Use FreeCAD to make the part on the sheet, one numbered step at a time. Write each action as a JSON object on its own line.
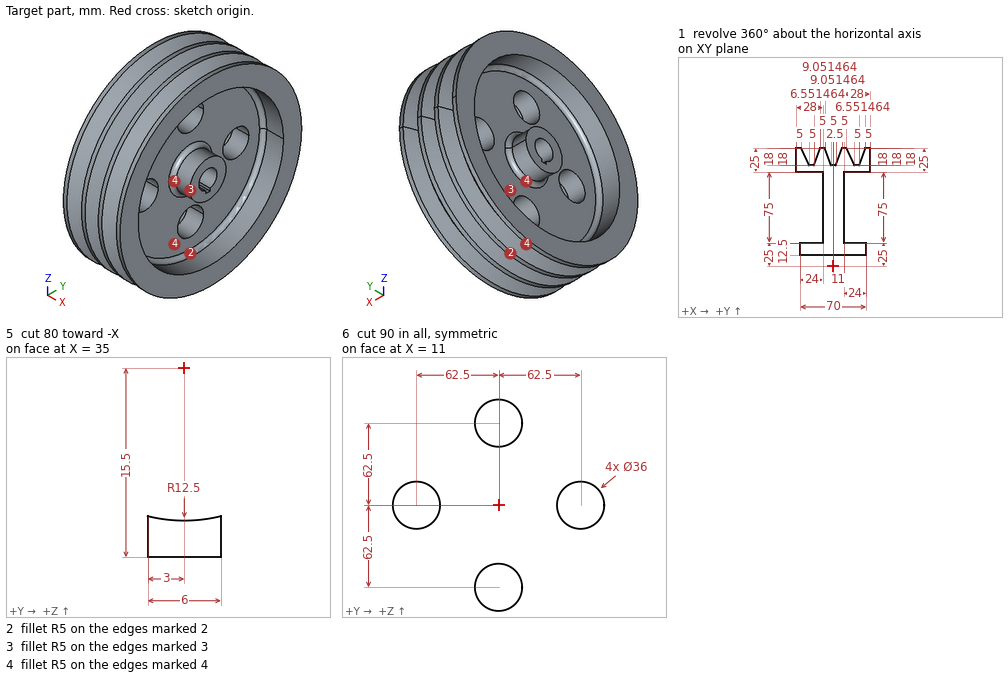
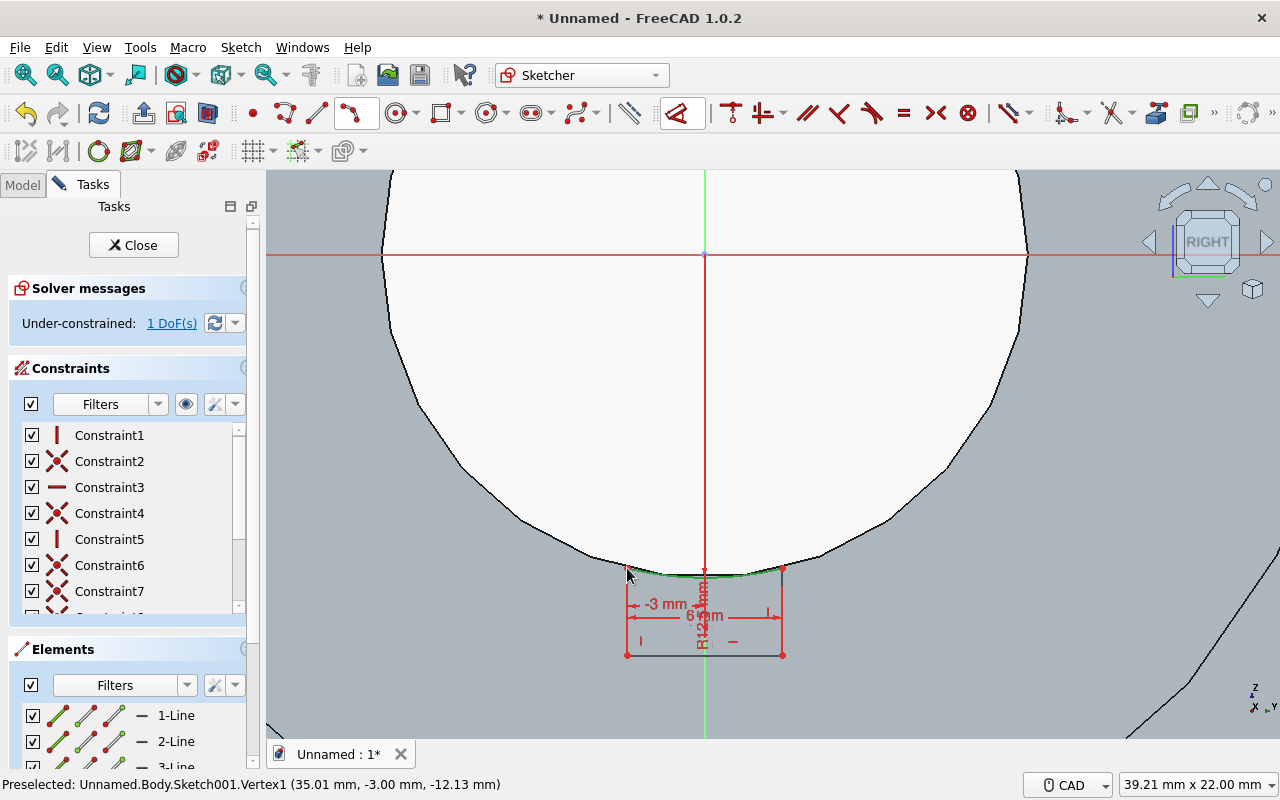
{"action": "left_click", "coordinate": [627, 656]}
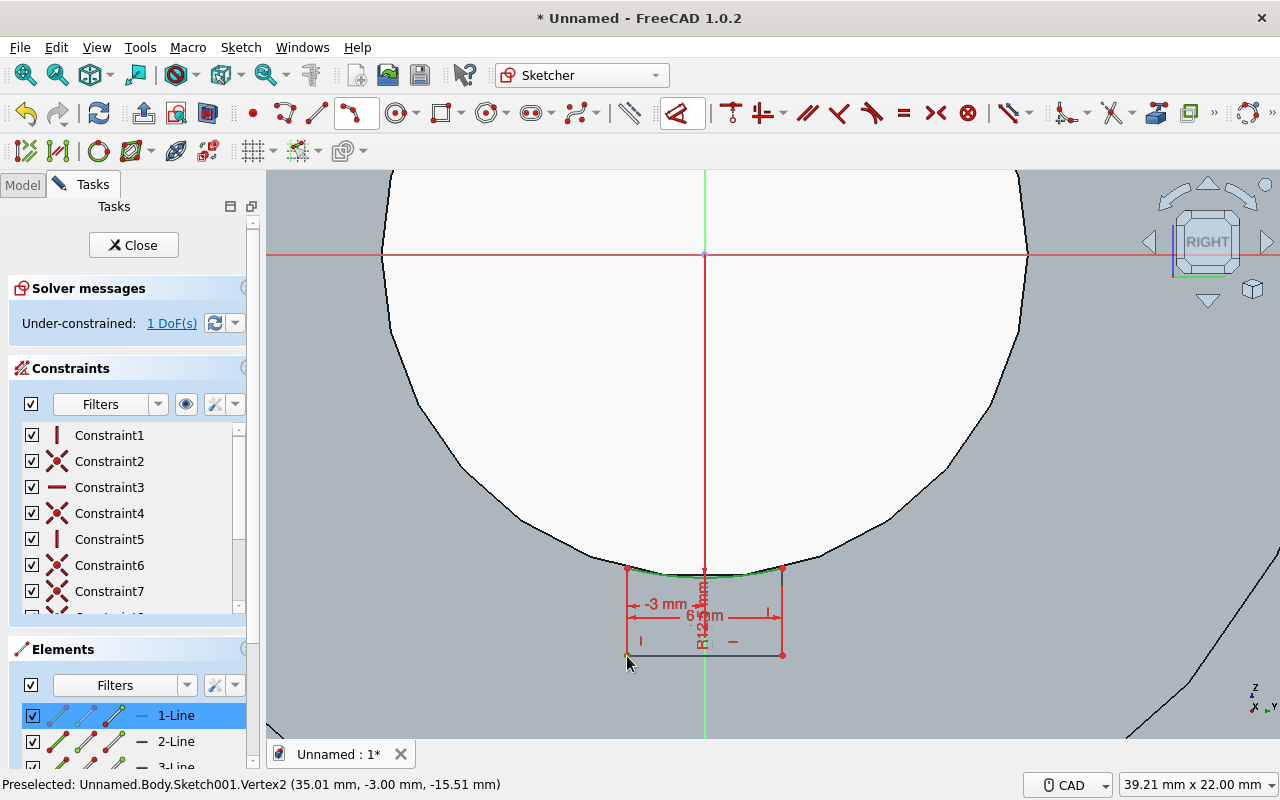
{"action": "left_click", "coordinate": [700, 114]}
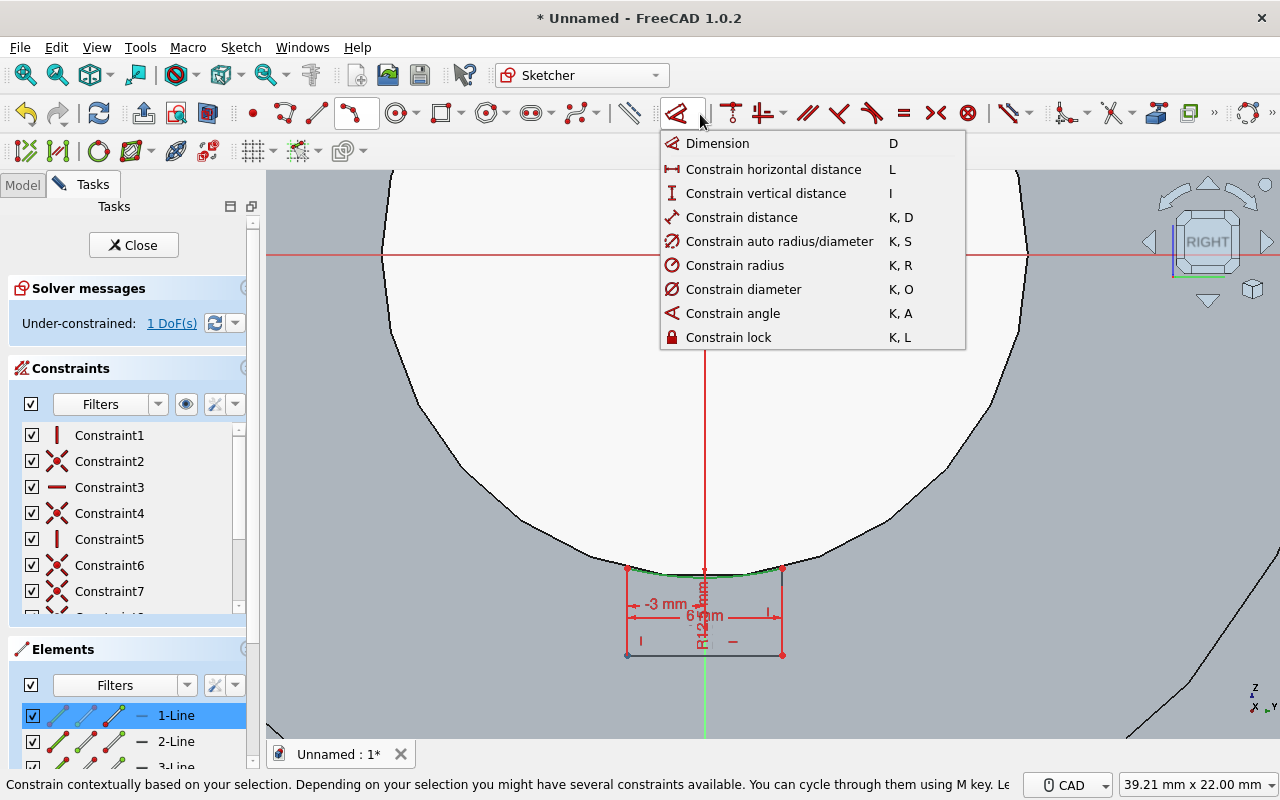
{"action": "left_click", "coordinate": [813, 193]}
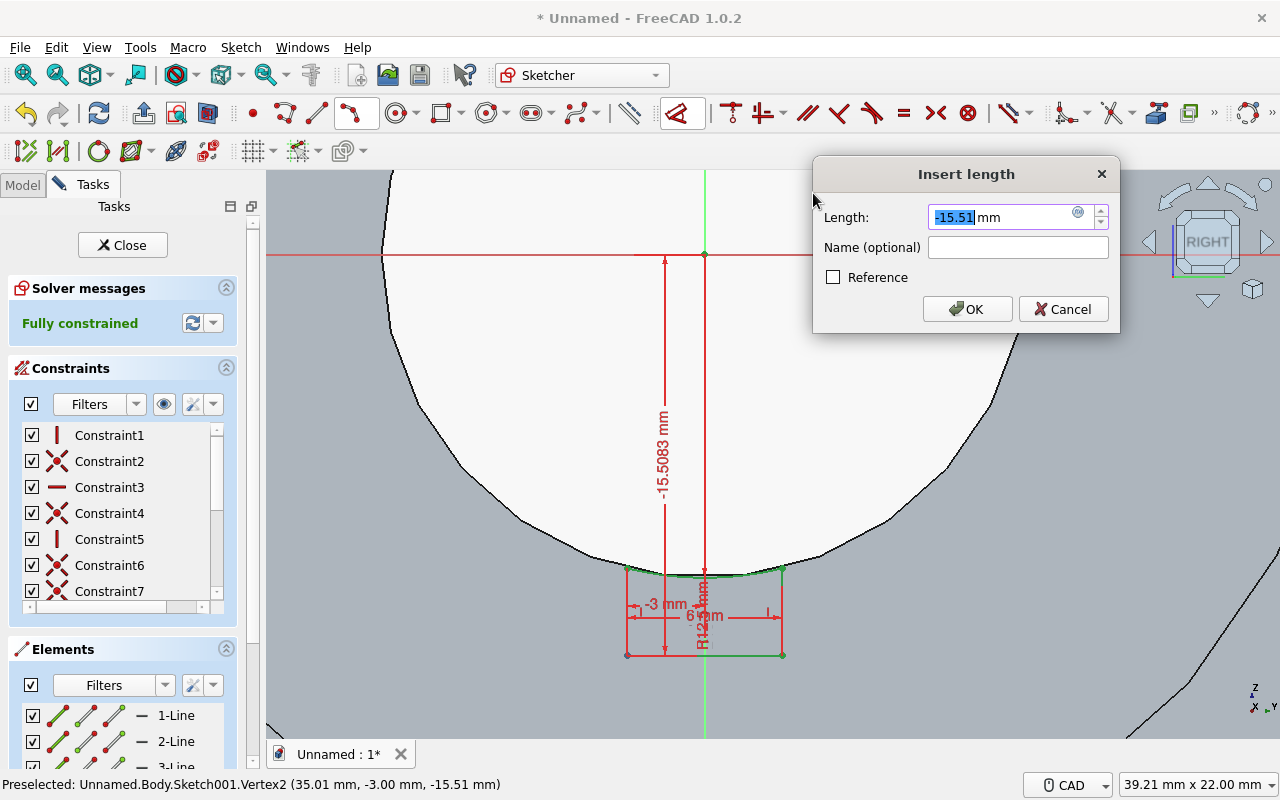
{"action": "type", "text": "-15.5"}
{"action": "key", "text": "Return"}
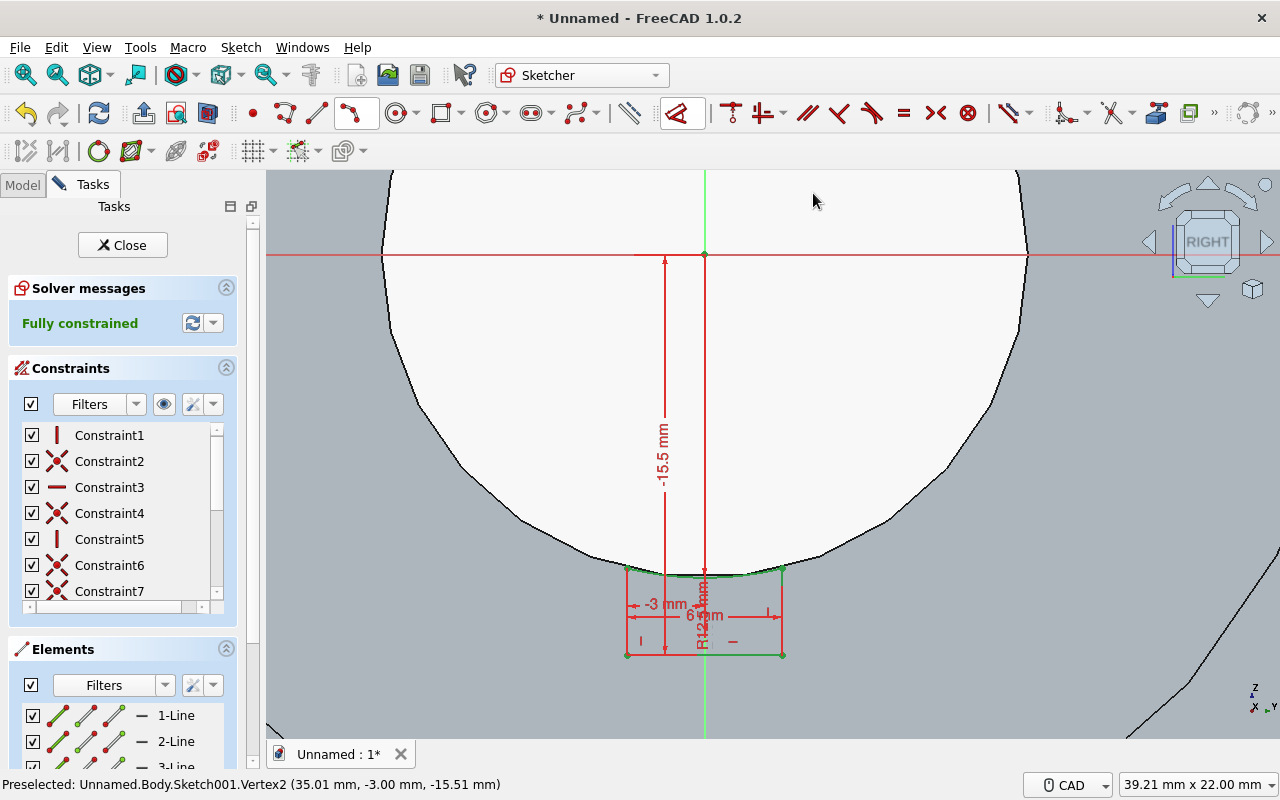
{"action": "left_click", "coordinate": [123, 245]}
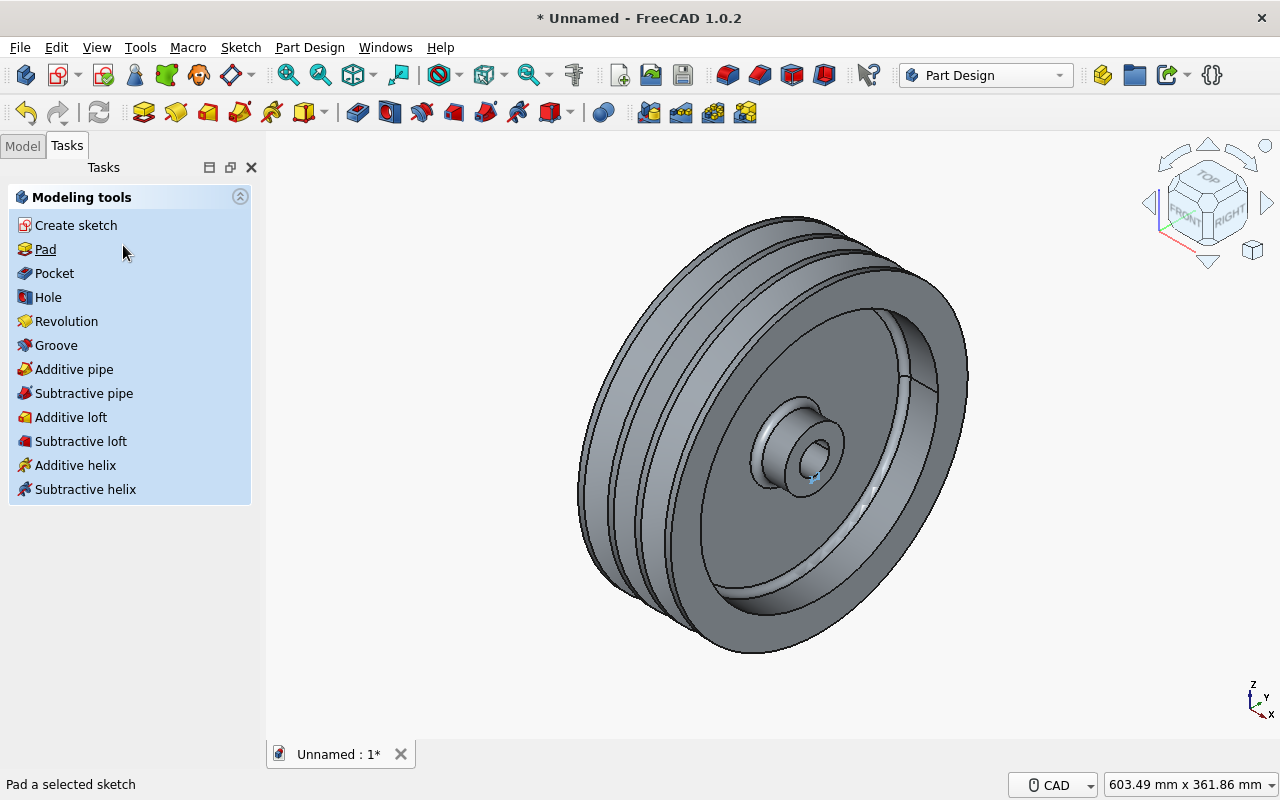
{"action": "left_click", "coordinate": [358, 112]}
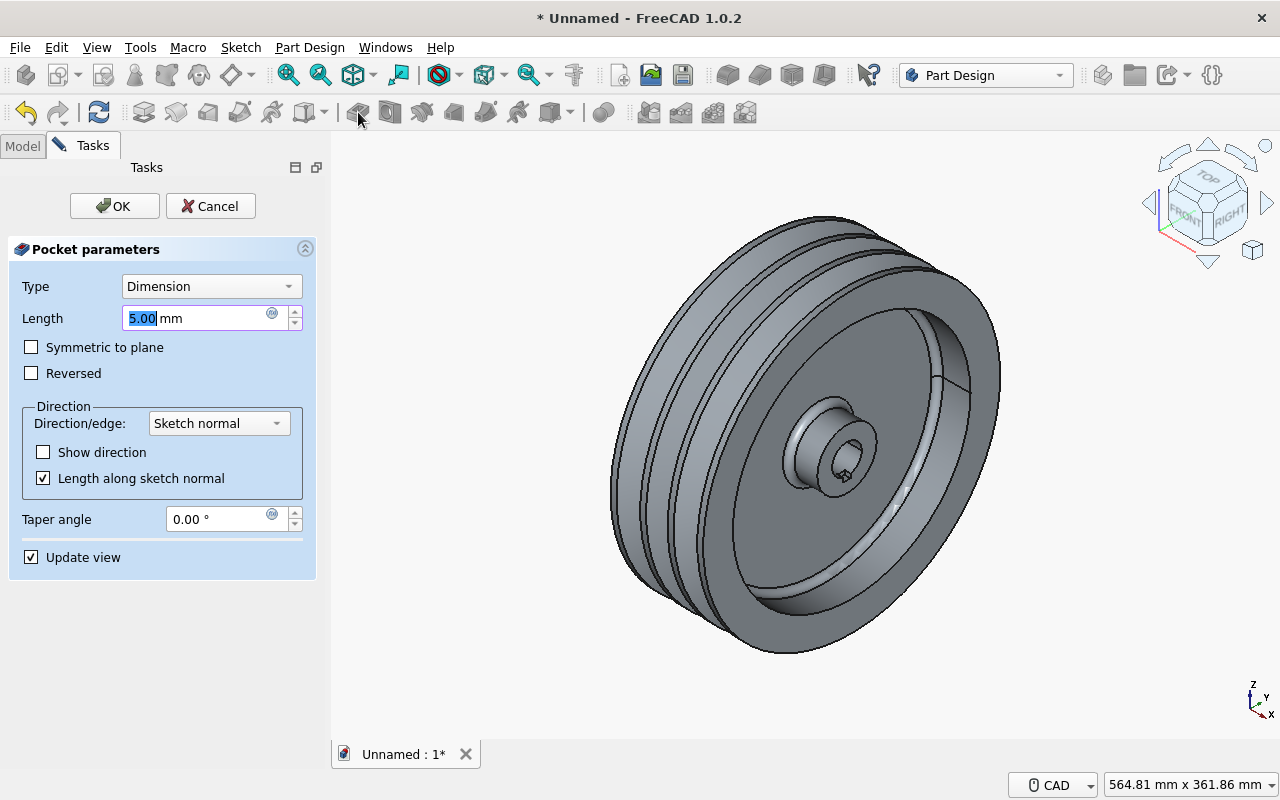
{"action": "type", "text": "80"}
{"action": "key", "text": "Tab"}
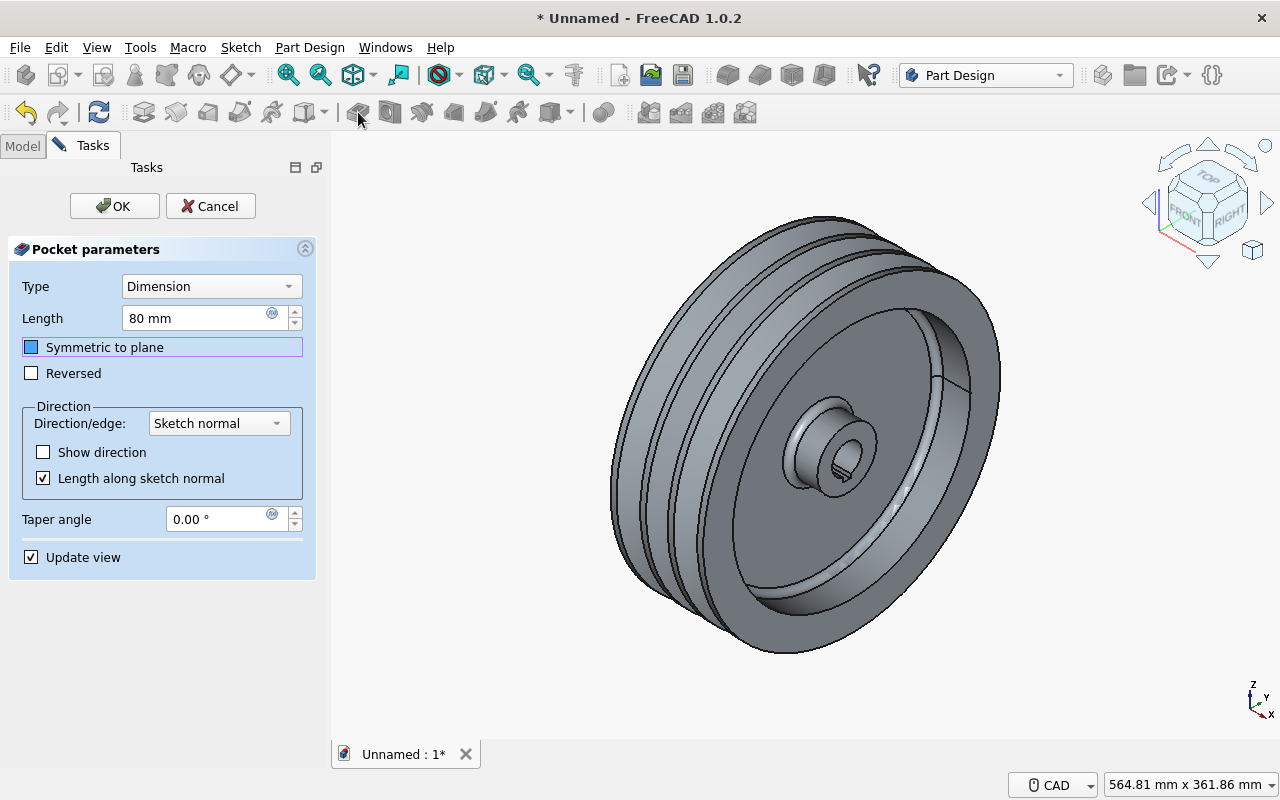
{"action": "left_click", "coordinate": [115, 206]}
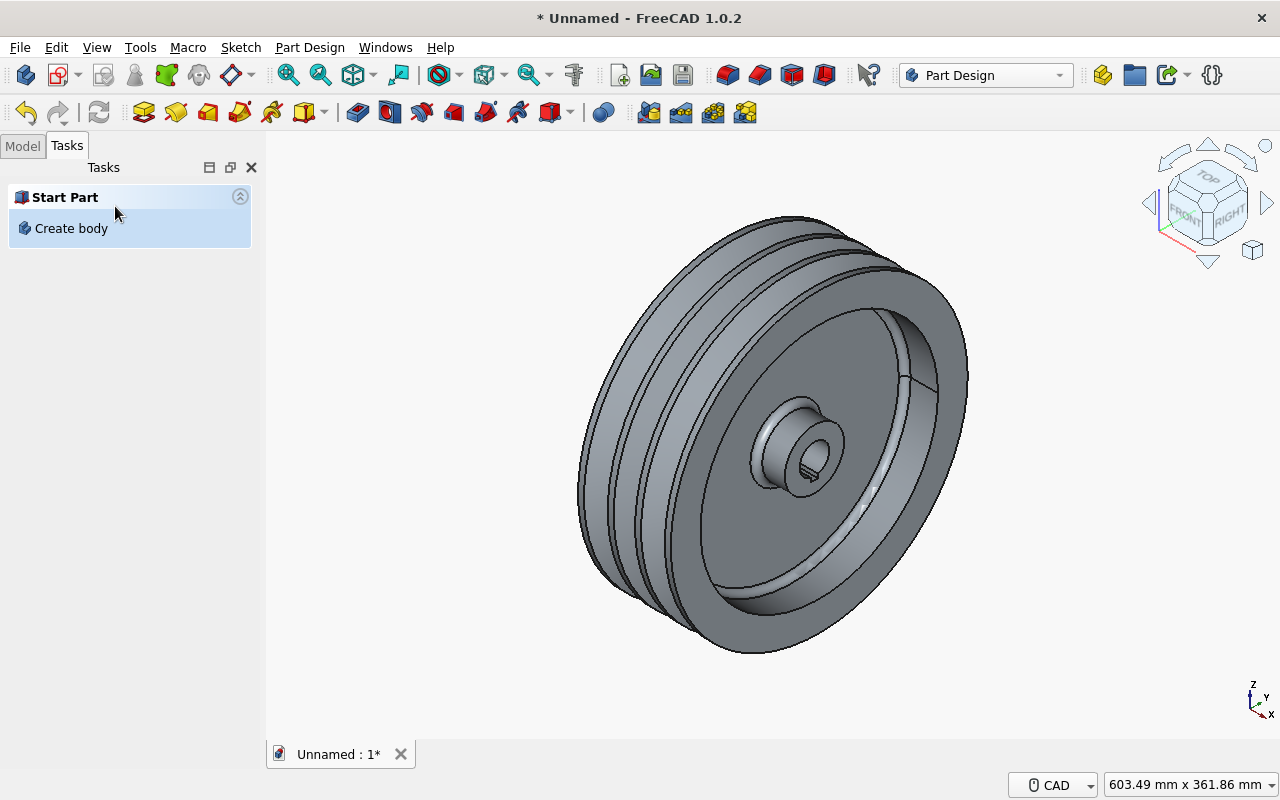
{"action": "left_click", "coordinate": [850, 367]}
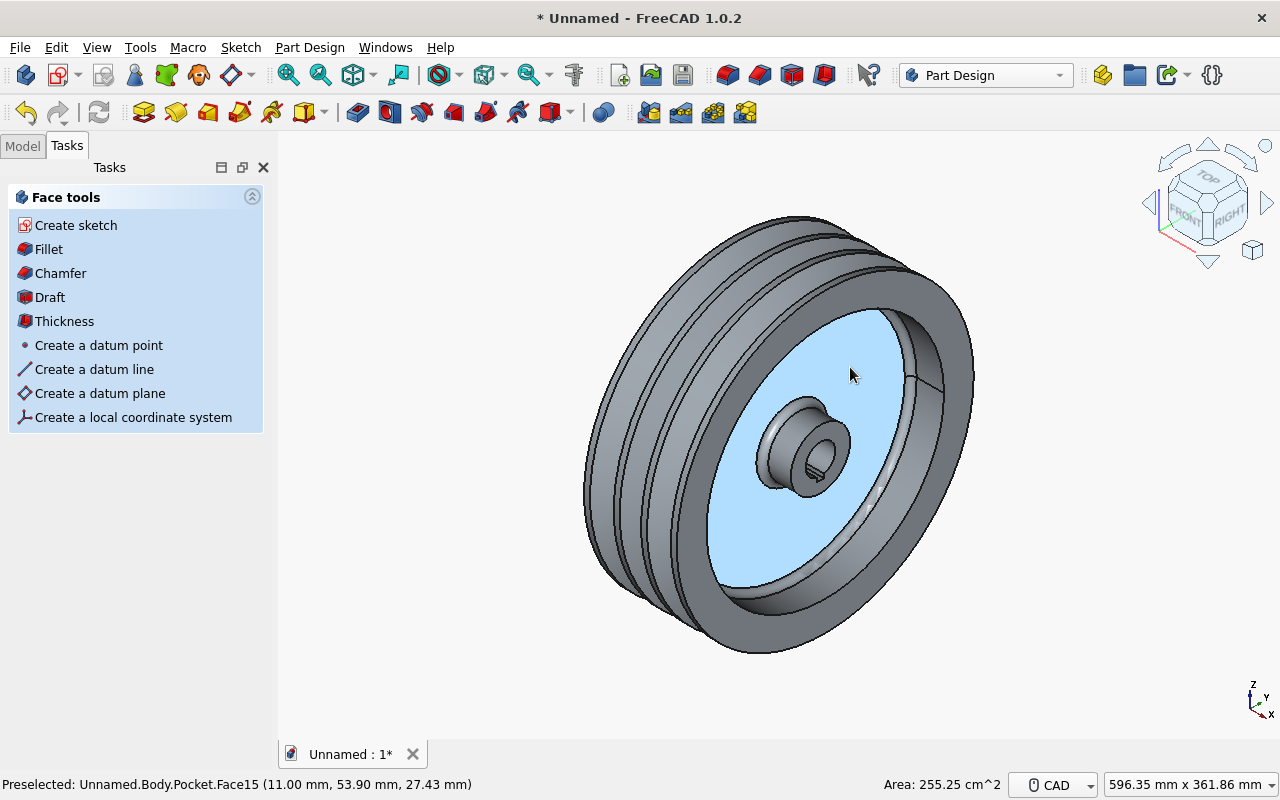
{"action": "left_click", "coordinate": [58, 76]}